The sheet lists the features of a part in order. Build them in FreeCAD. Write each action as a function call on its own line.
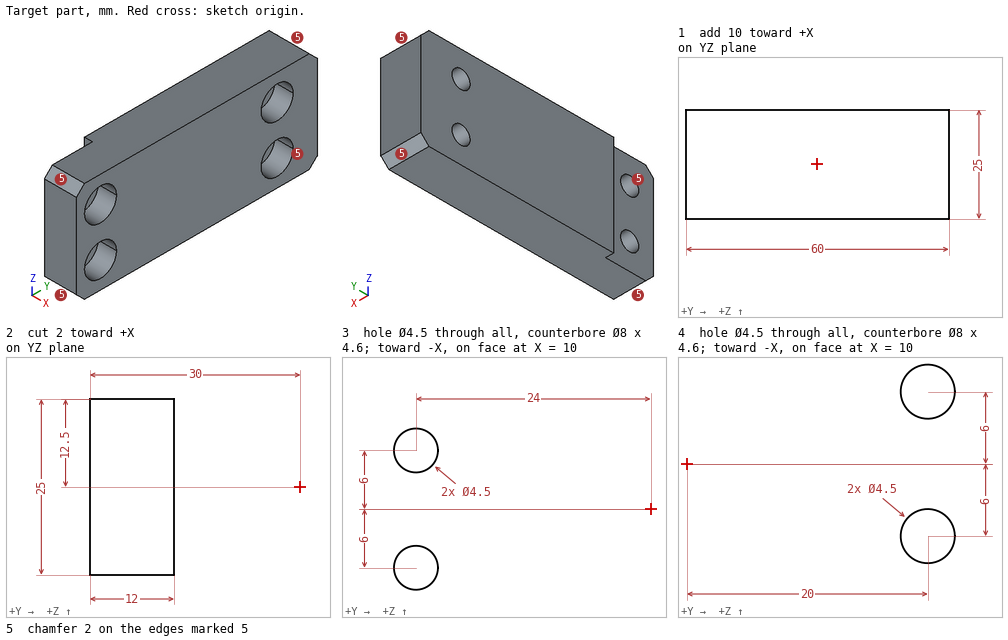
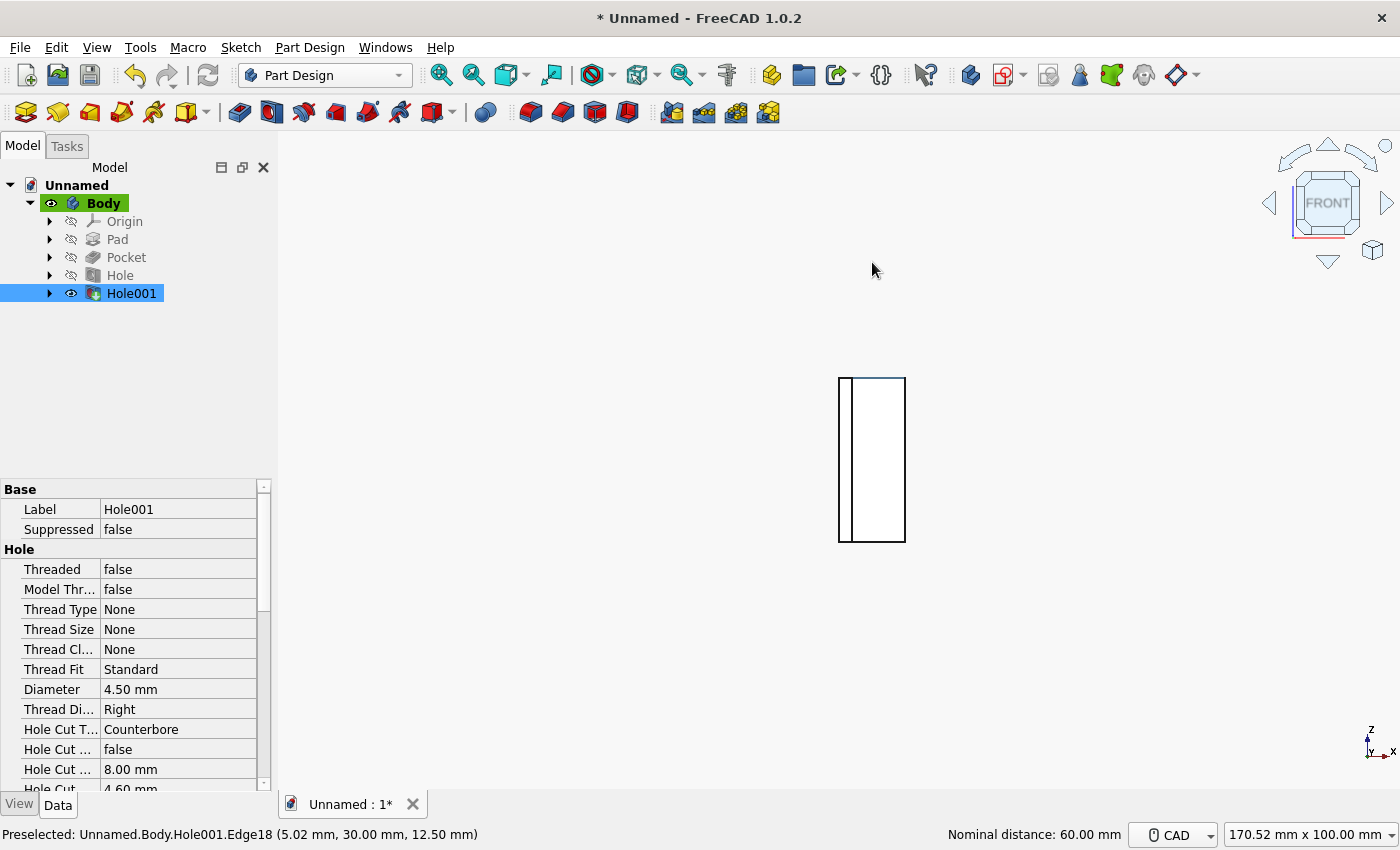
key(v)
key(f)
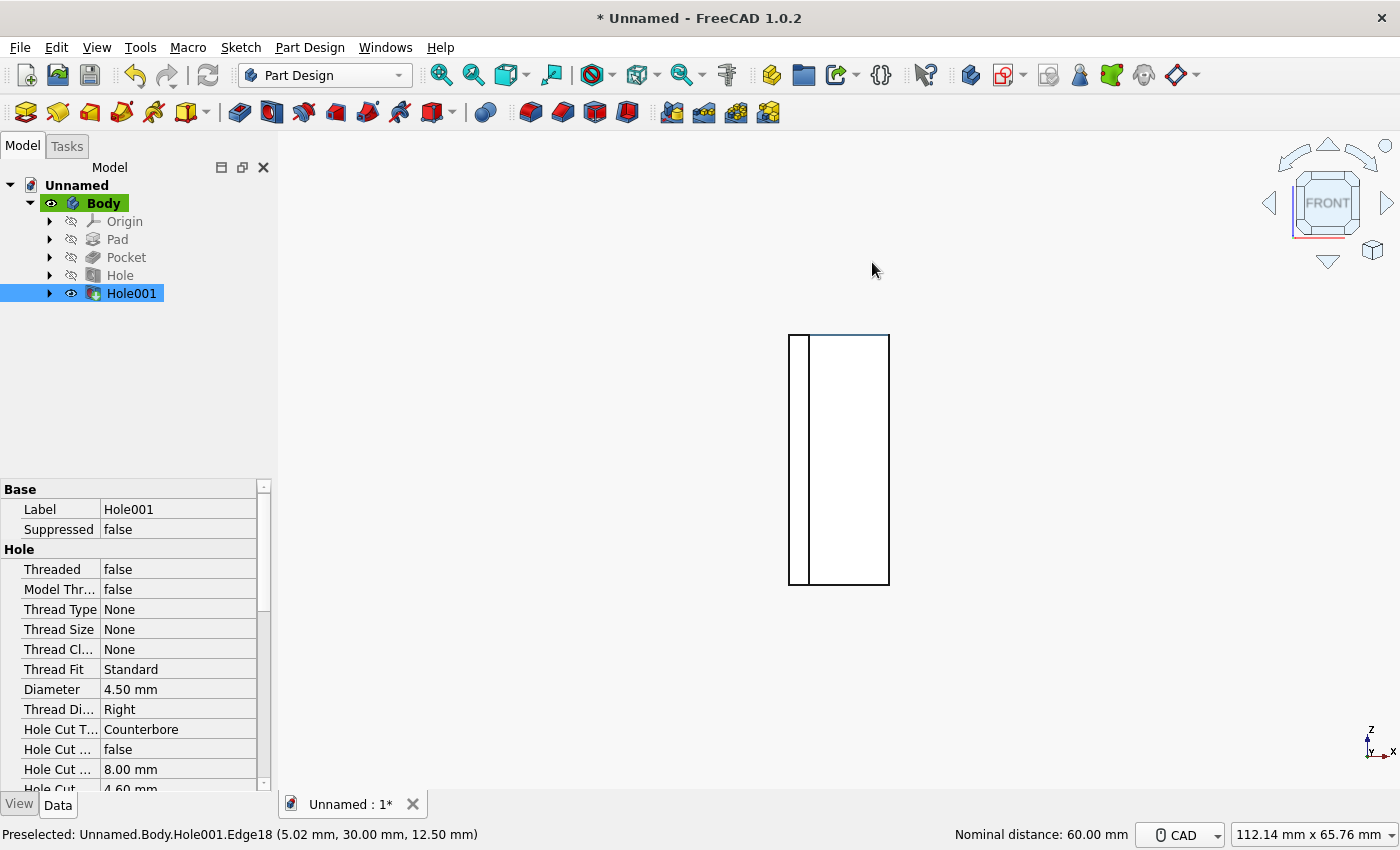
click(849, 584, ctrl)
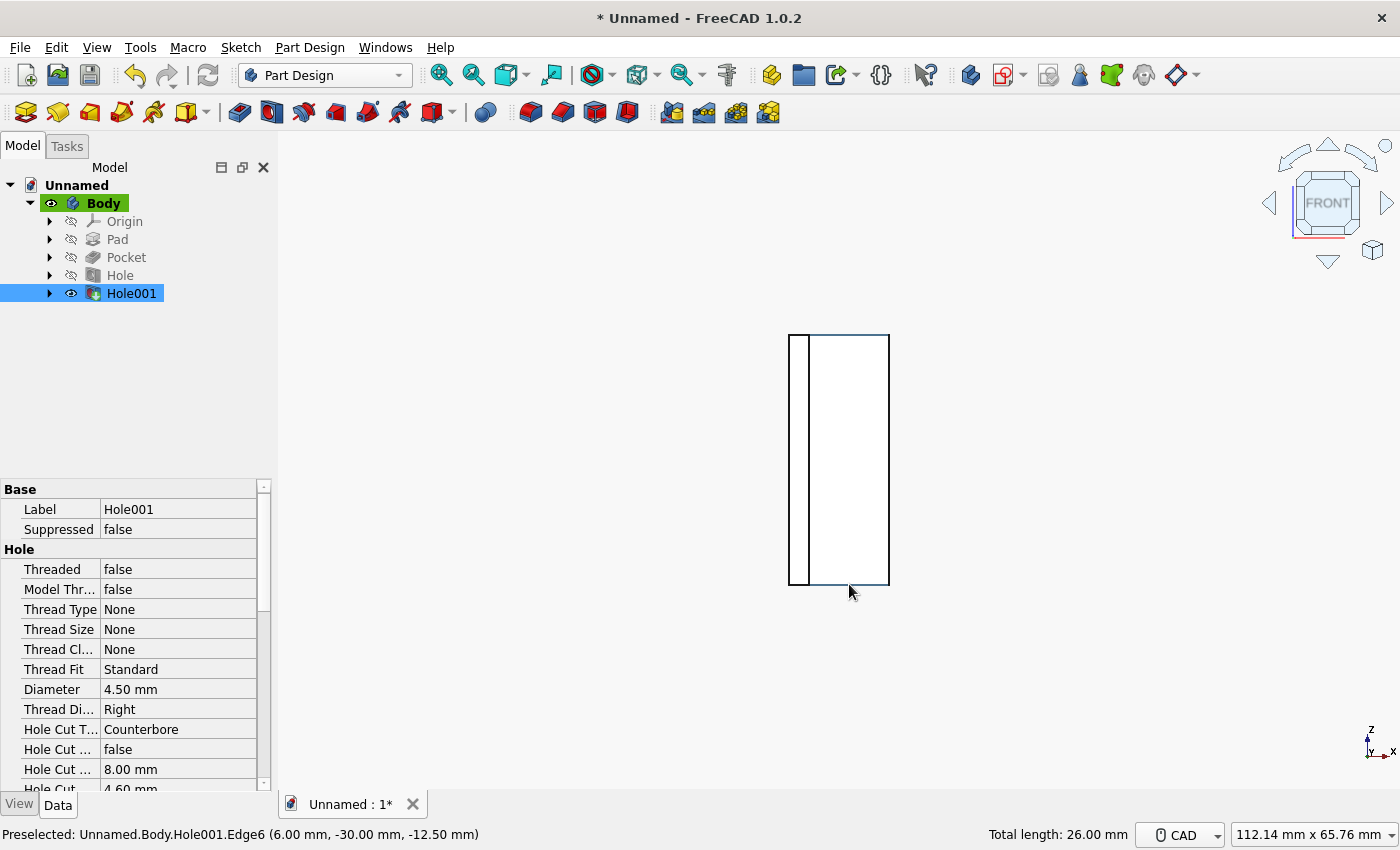
key(3)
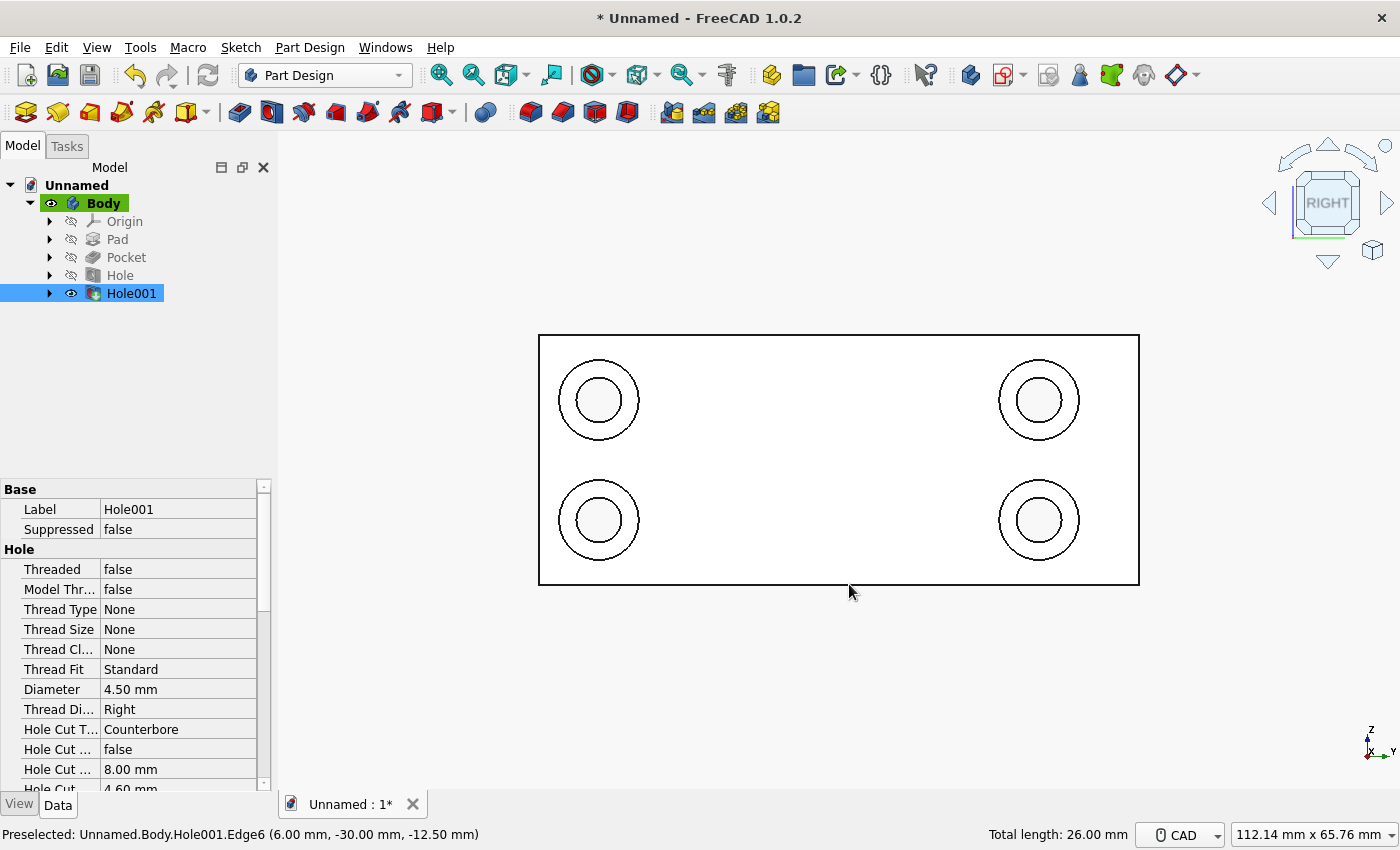
key(5)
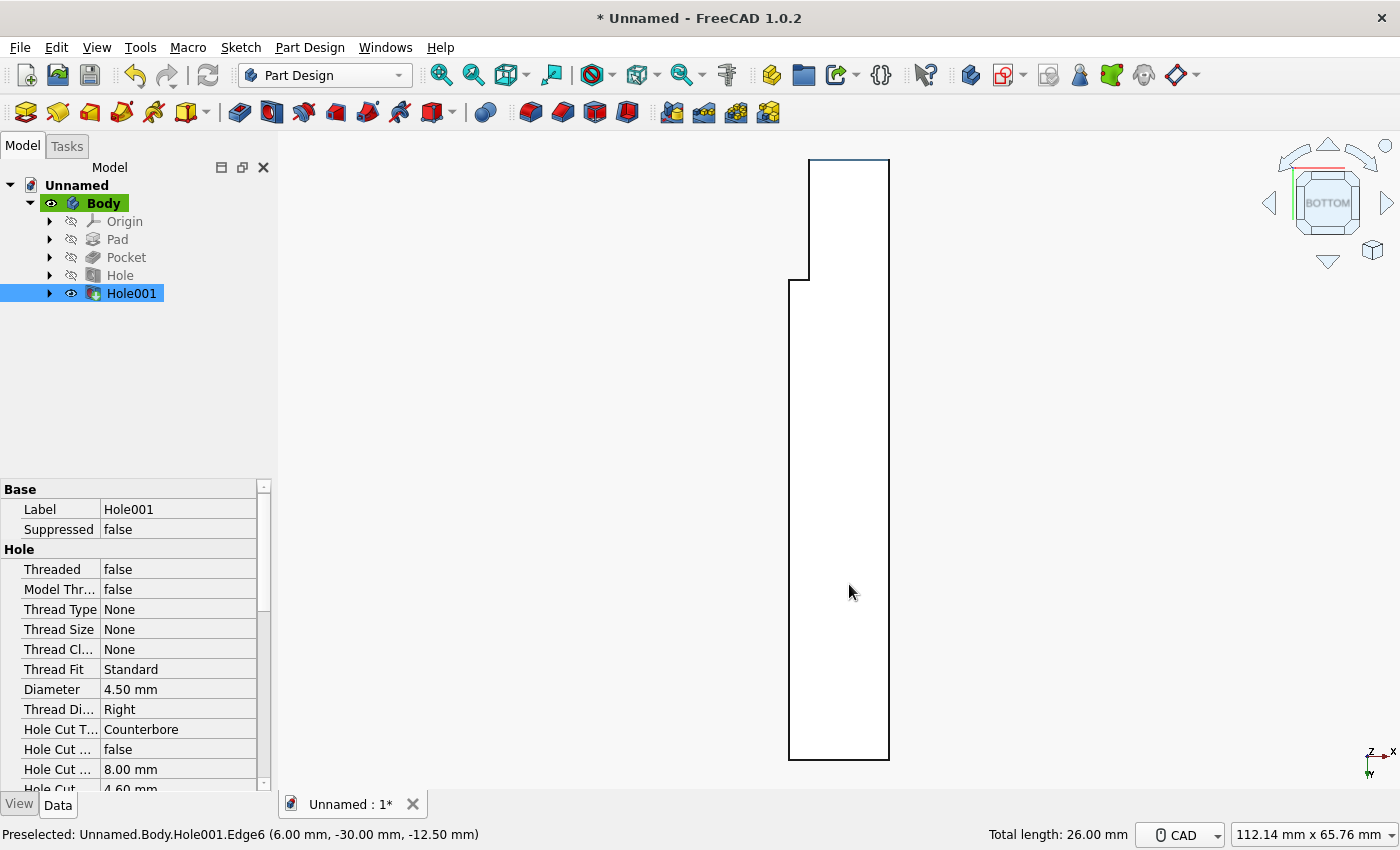
click(839, 759, ctrl)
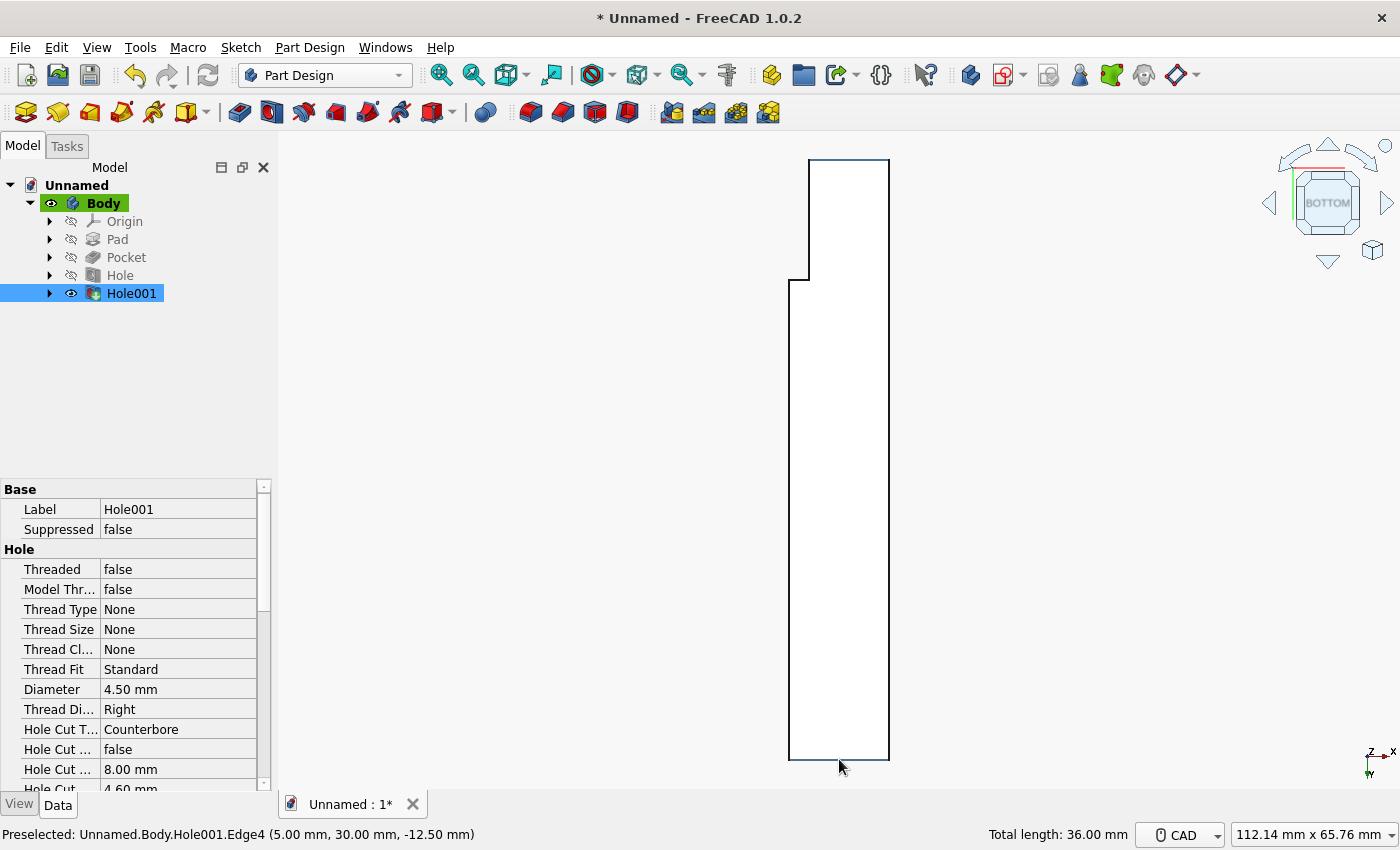
click(564, 112)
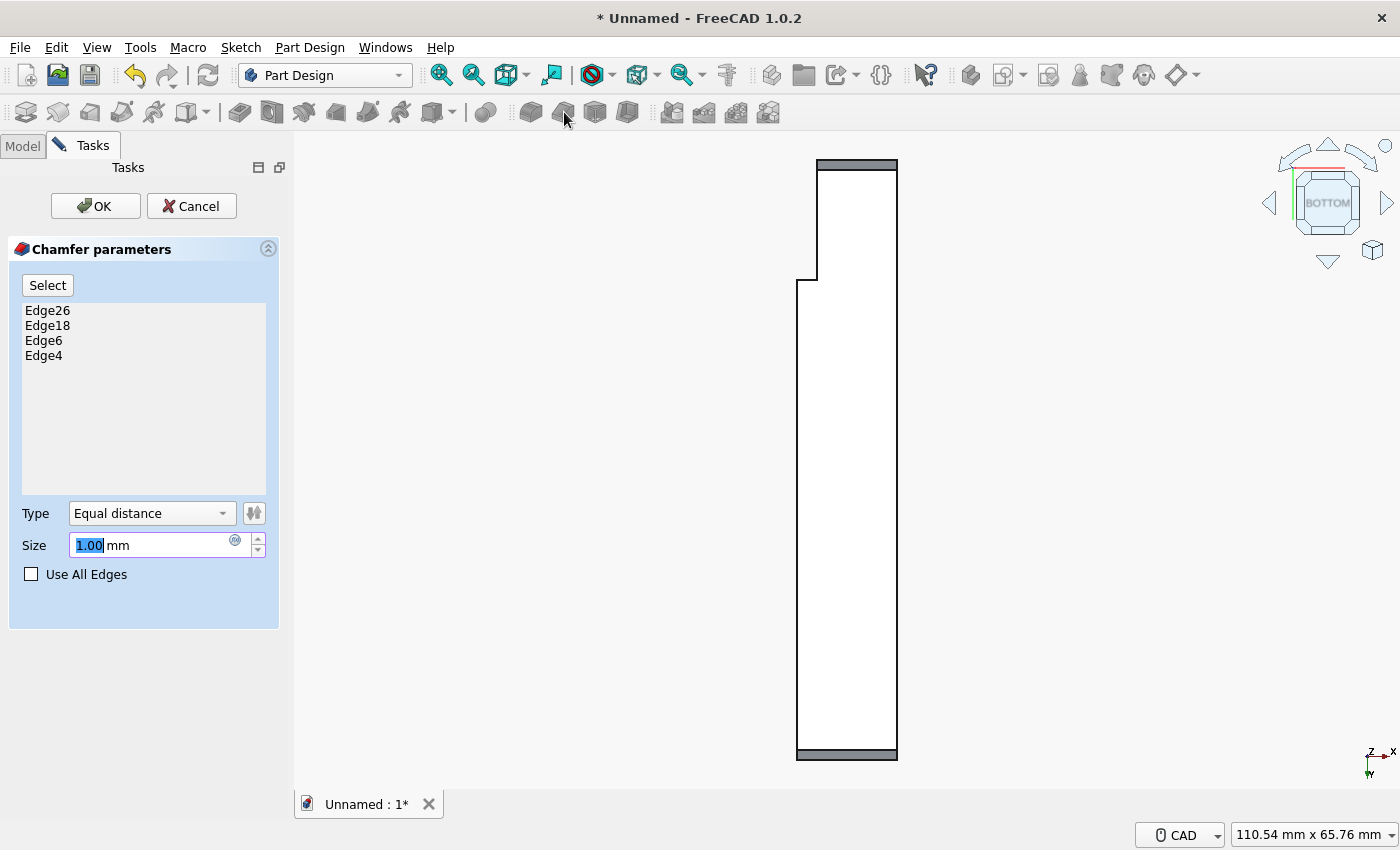
text(2)
key(Tab)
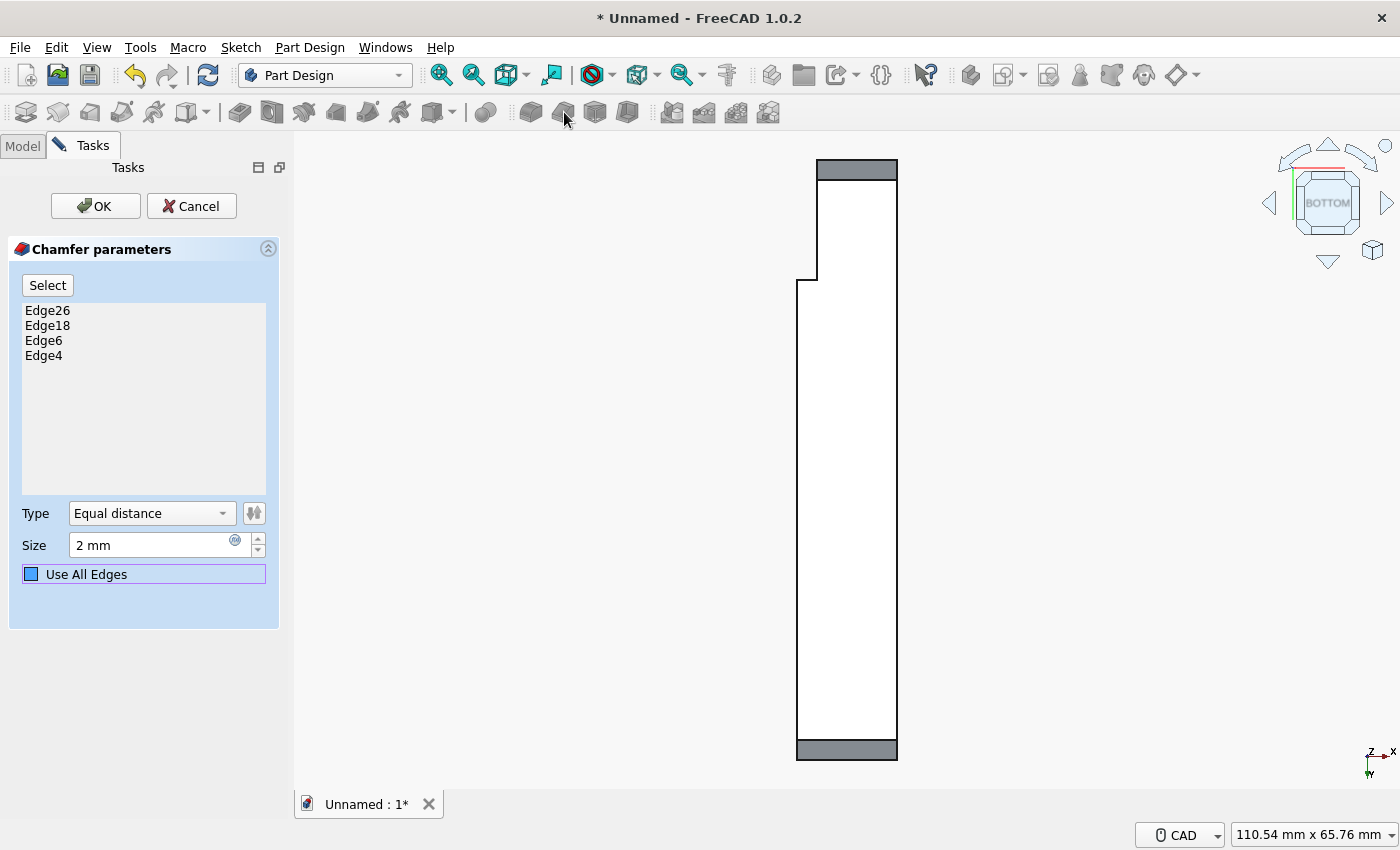
click(96, 206)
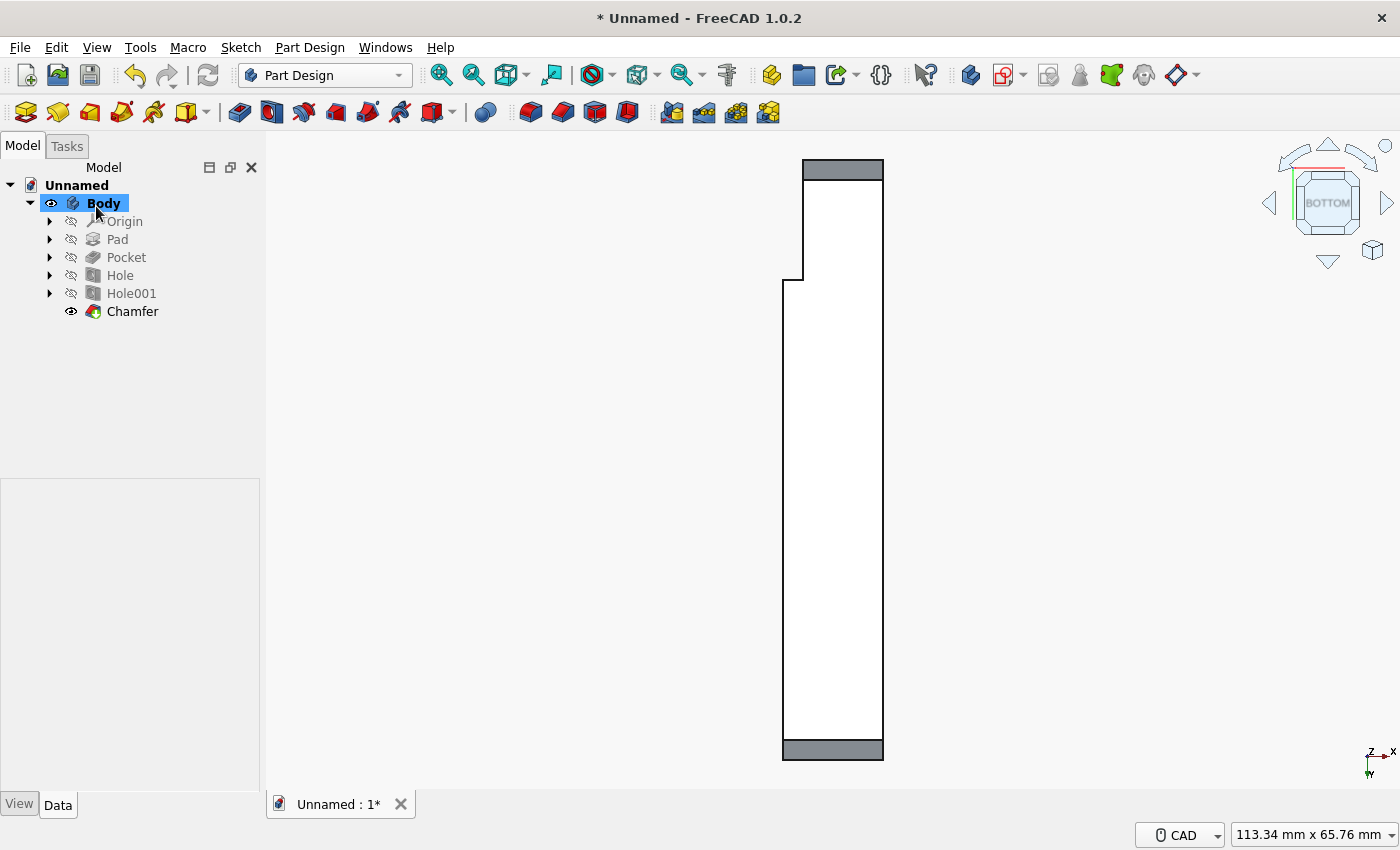
key(0)